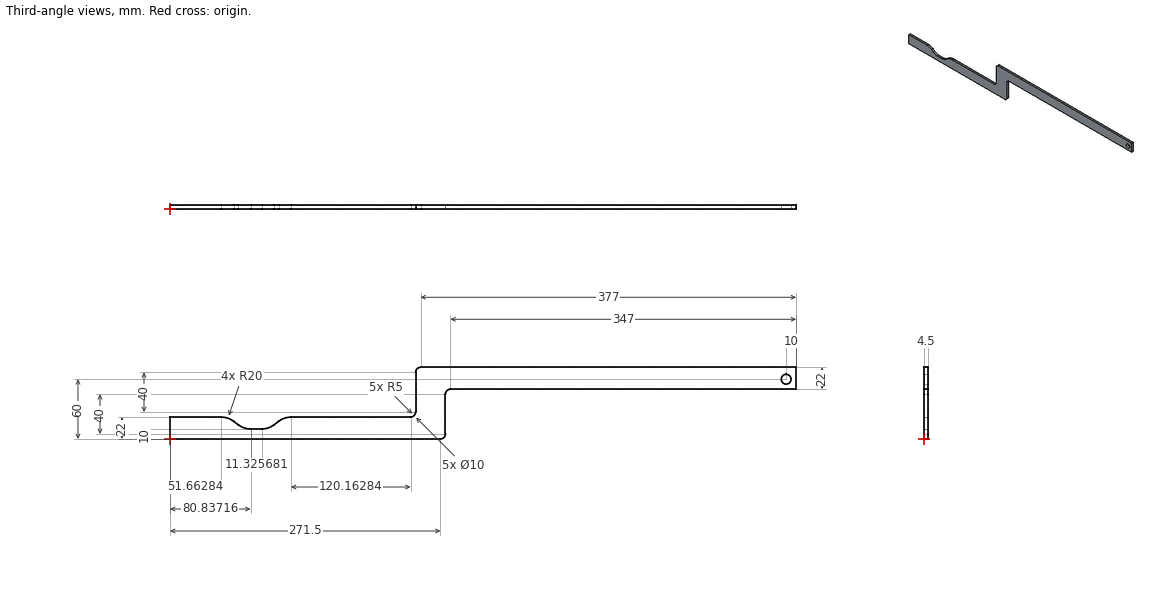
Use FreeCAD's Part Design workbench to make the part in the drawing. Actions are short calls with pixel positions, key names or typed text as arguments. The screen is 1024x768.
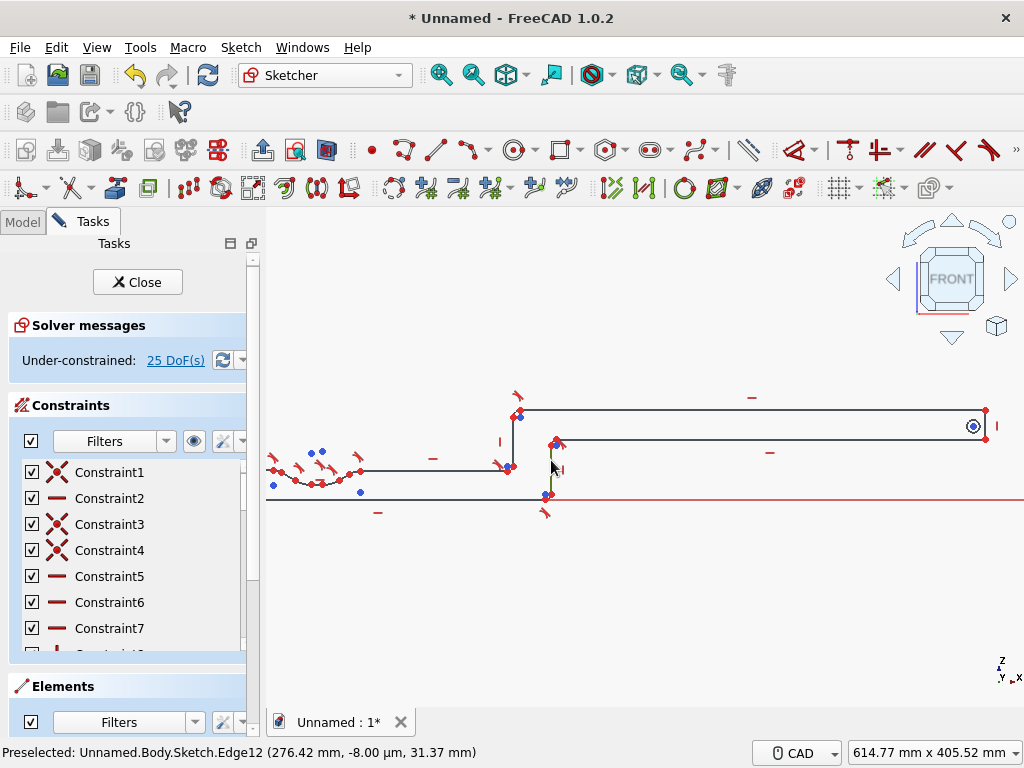
scroll(550, 498, up, 6)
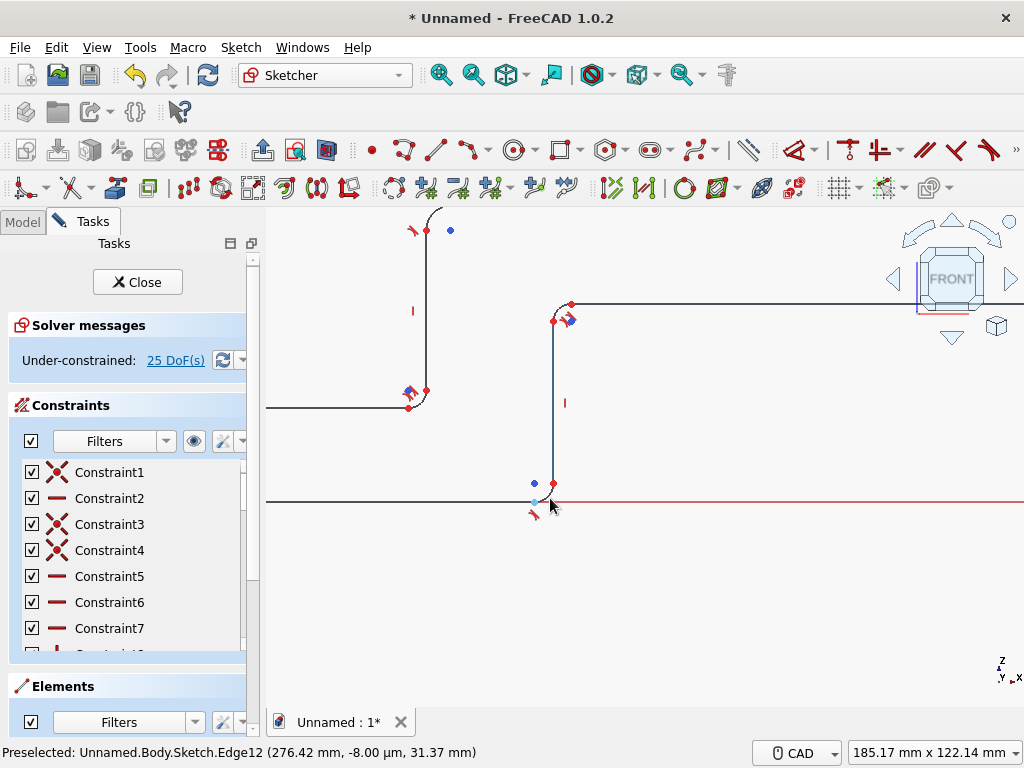
click(548, 497)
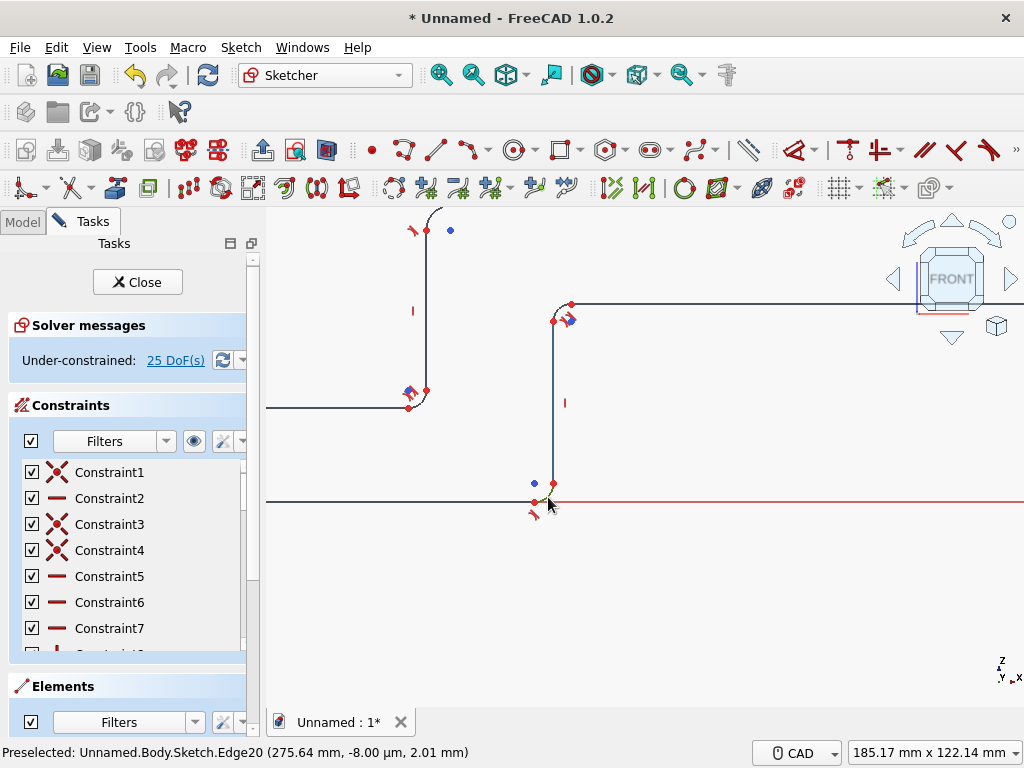
key(t)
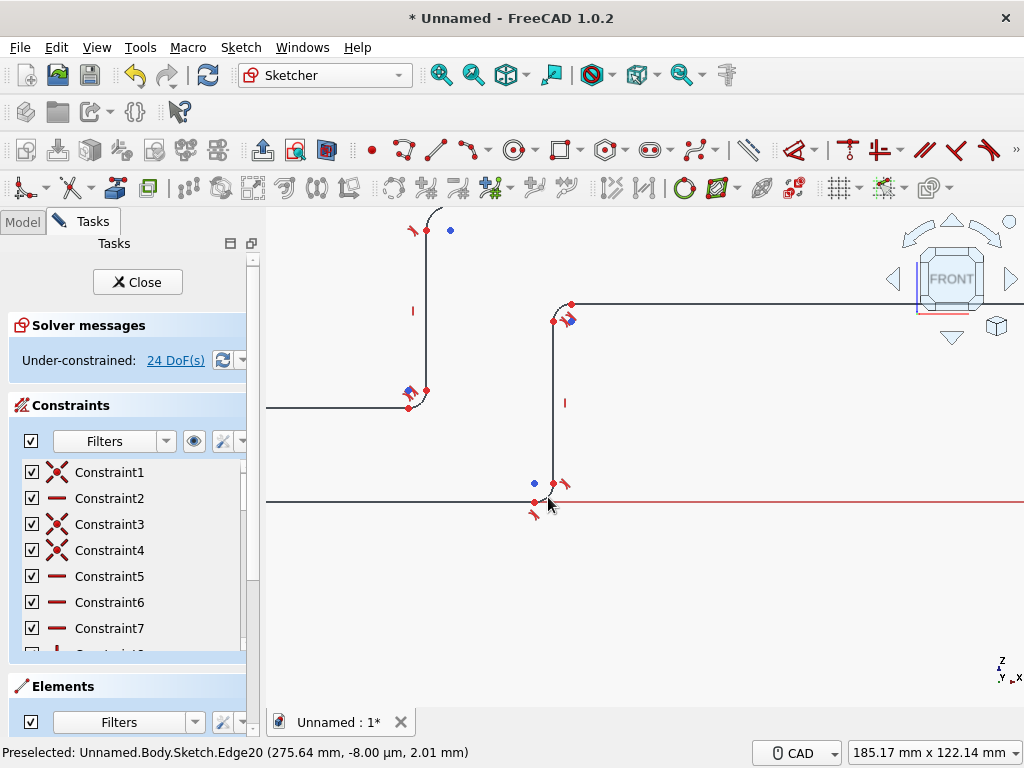
scroll(550, 477, down, 9)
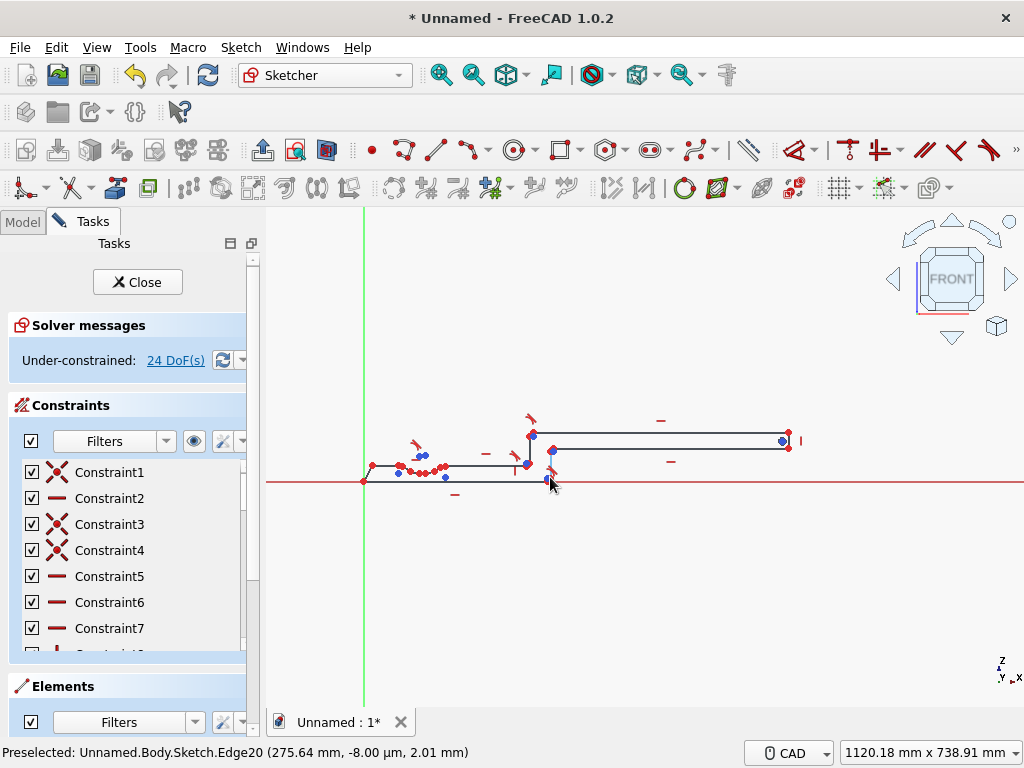
scroll(366, 477, up, 9)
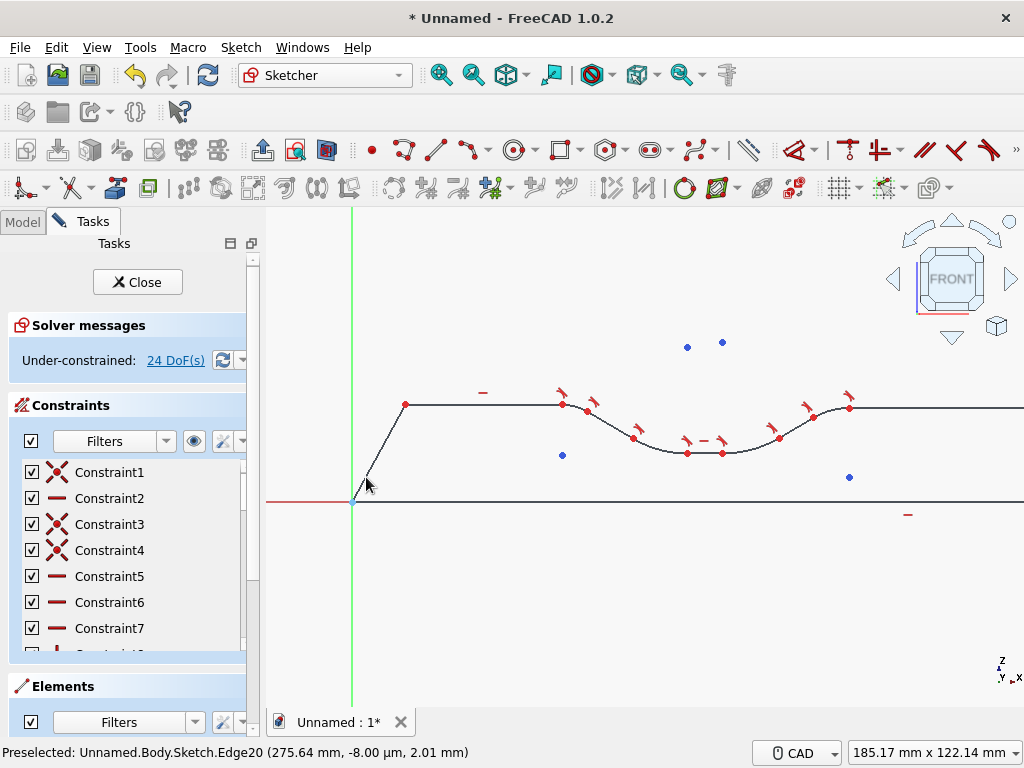
click(368, 473)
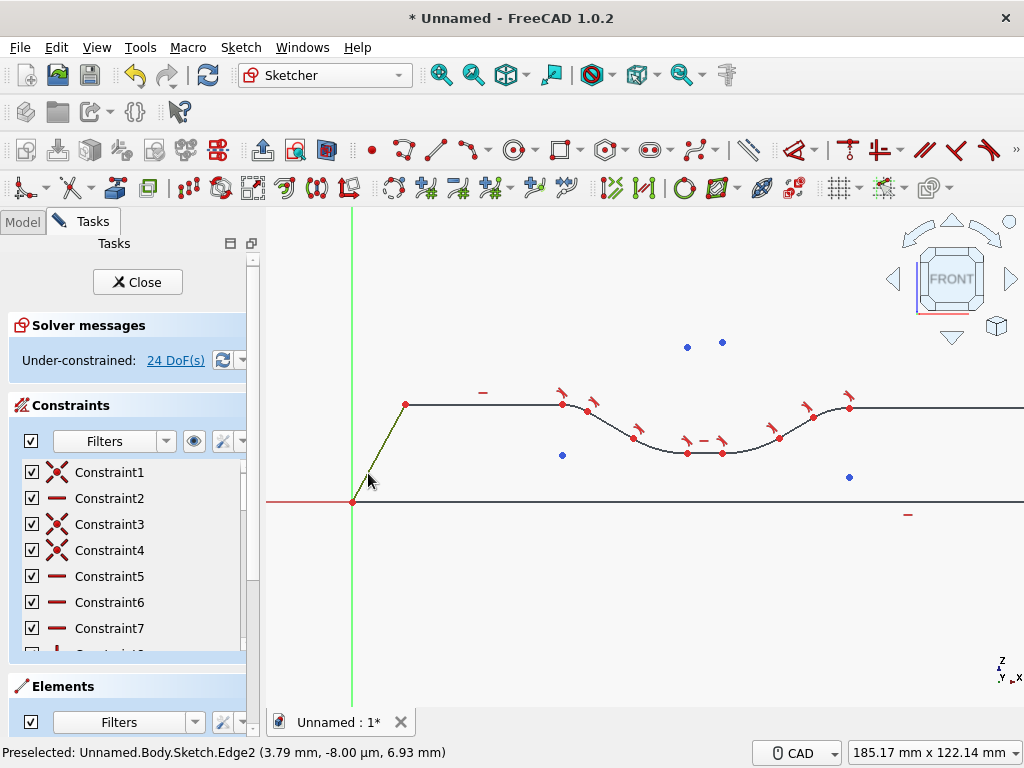
key(v)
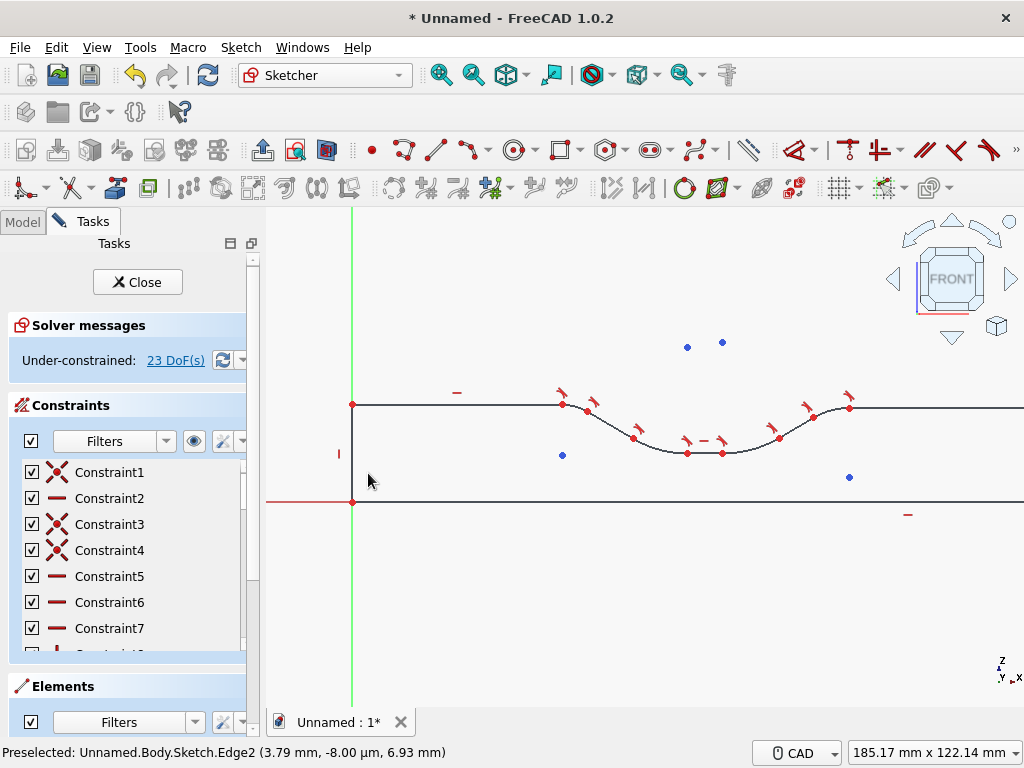
click(575, 407)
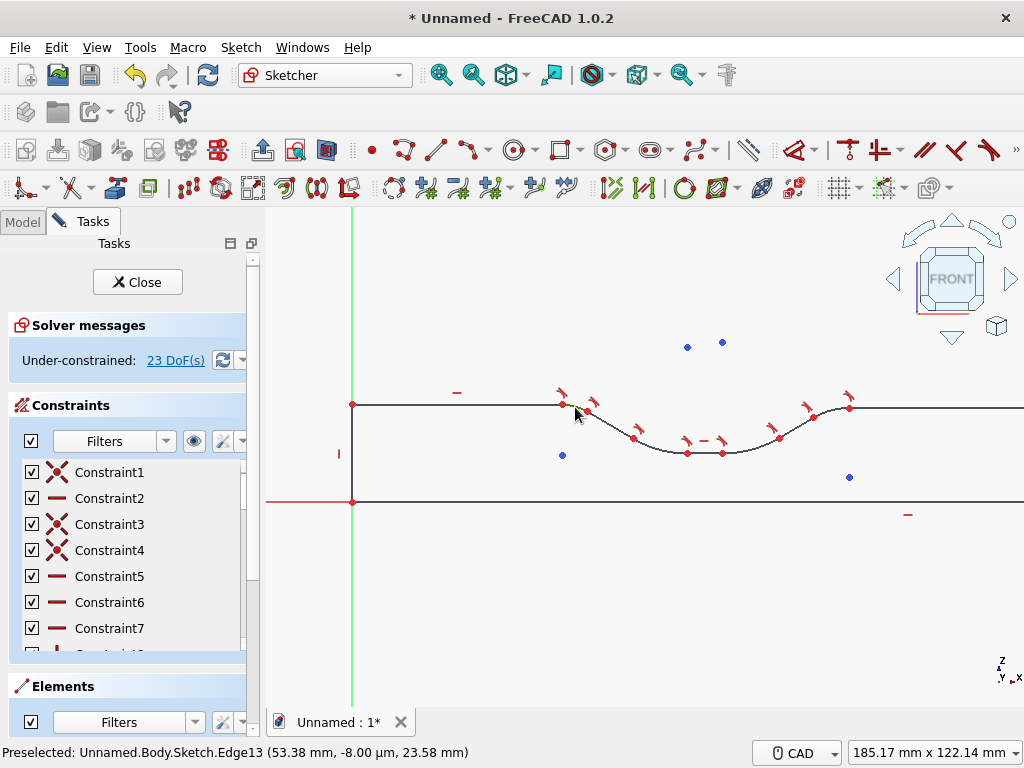
click(649, 446)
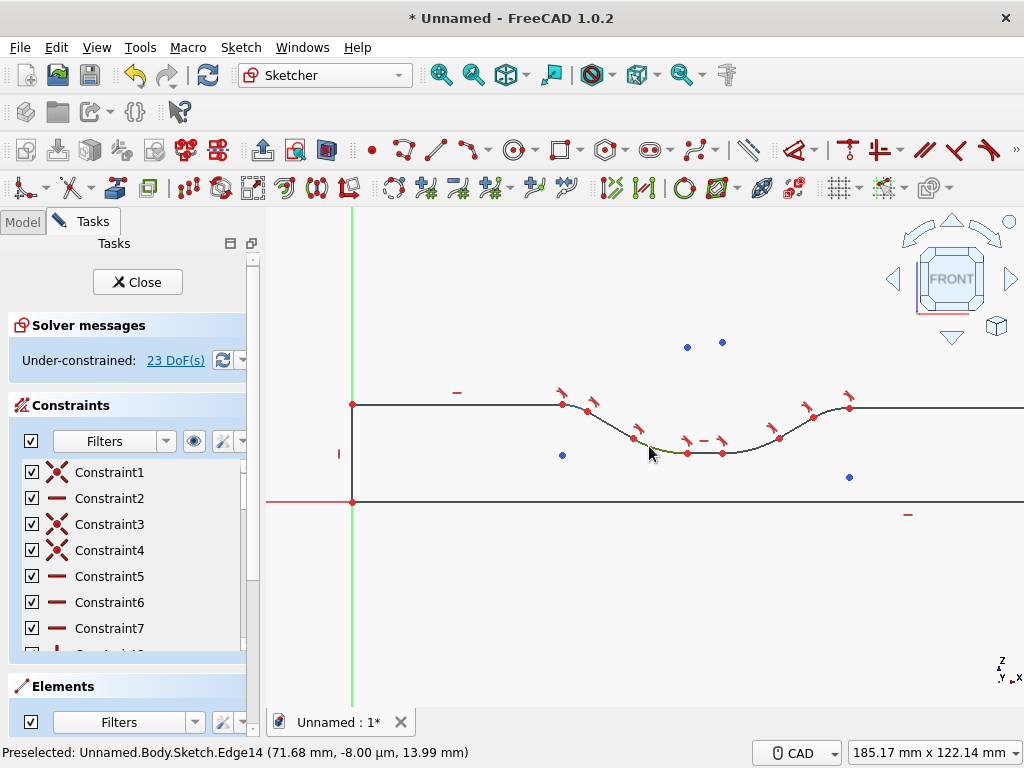
click(740, 452)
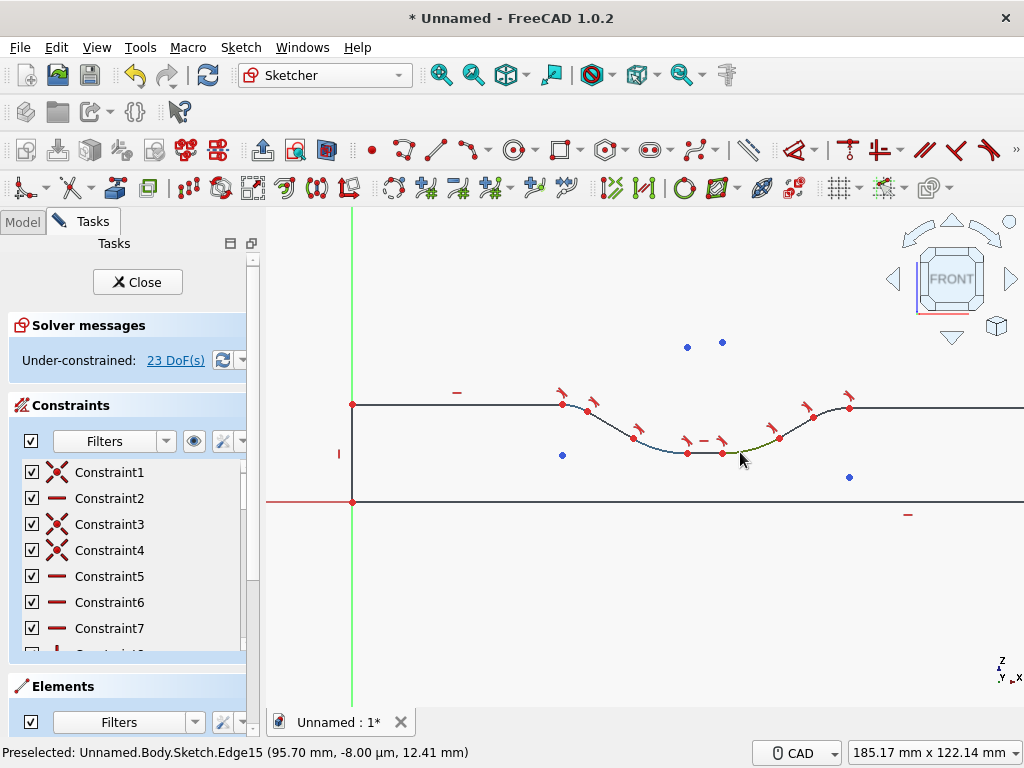
scroll(838, 409, up, 2)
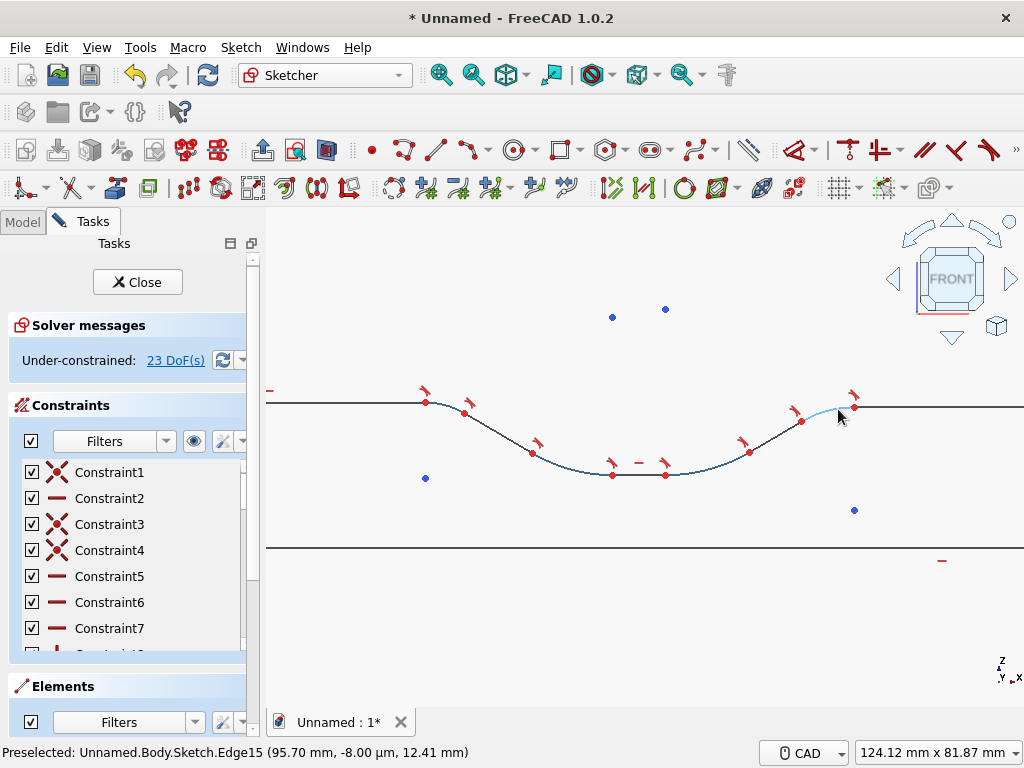
click(838, 409)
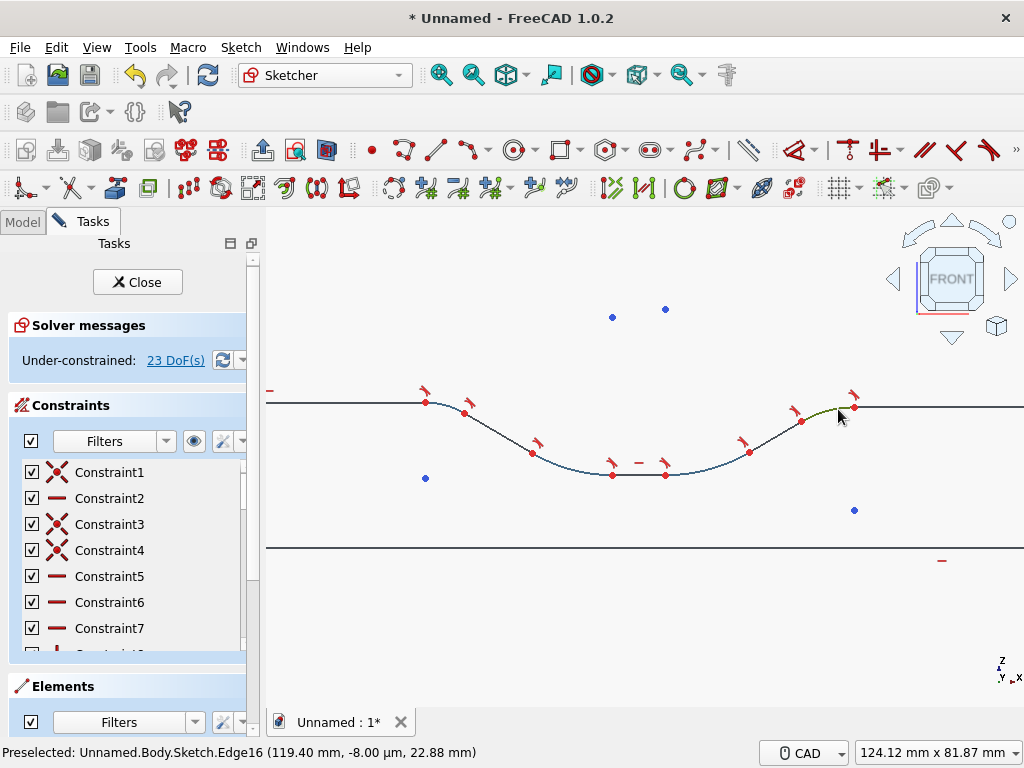
key(e)